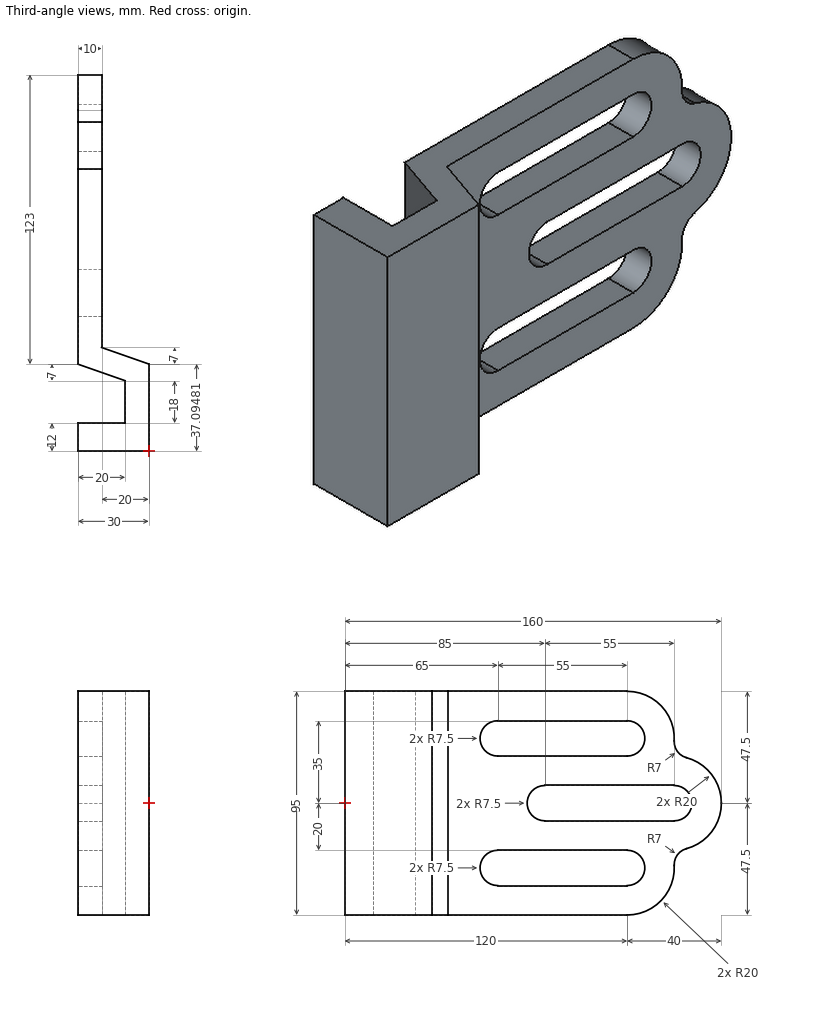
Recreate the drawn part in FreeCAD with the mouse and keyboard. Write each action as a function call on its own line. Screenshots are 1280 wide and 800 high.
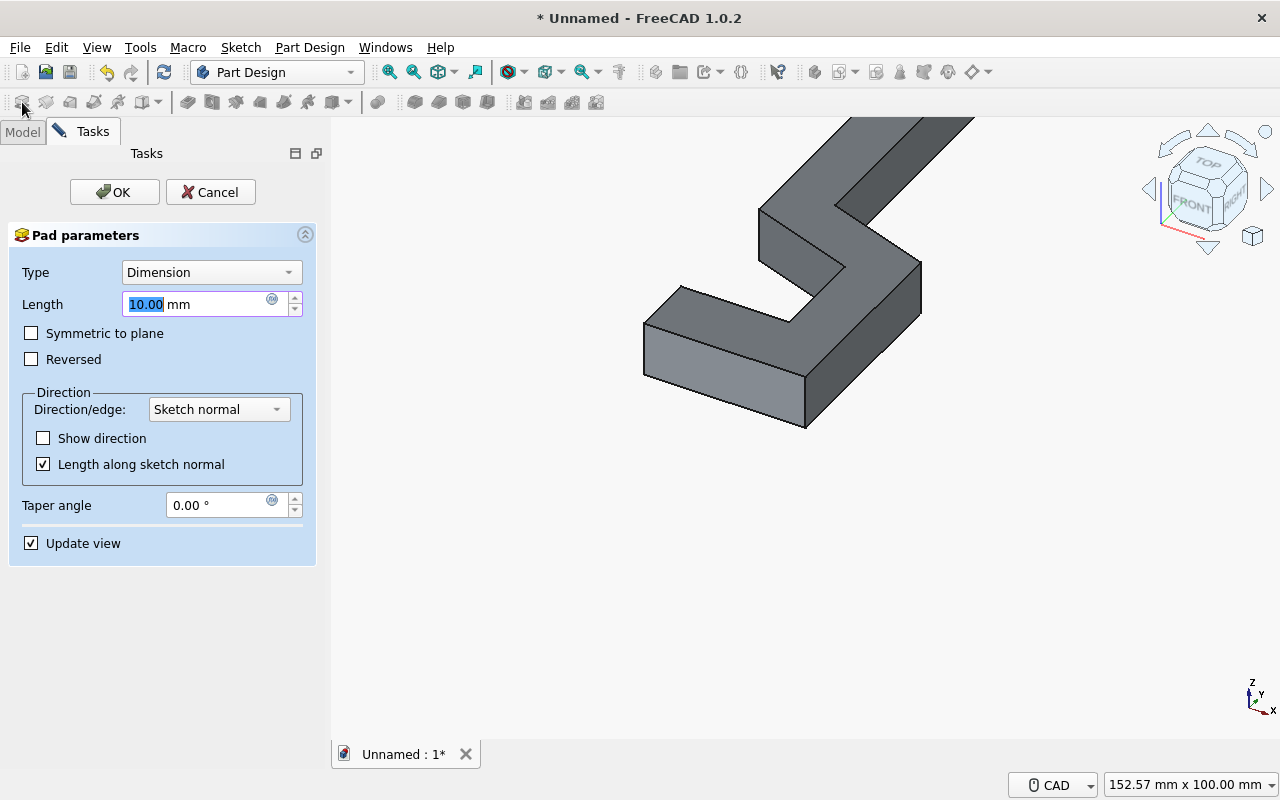
text(95)
key(Tab)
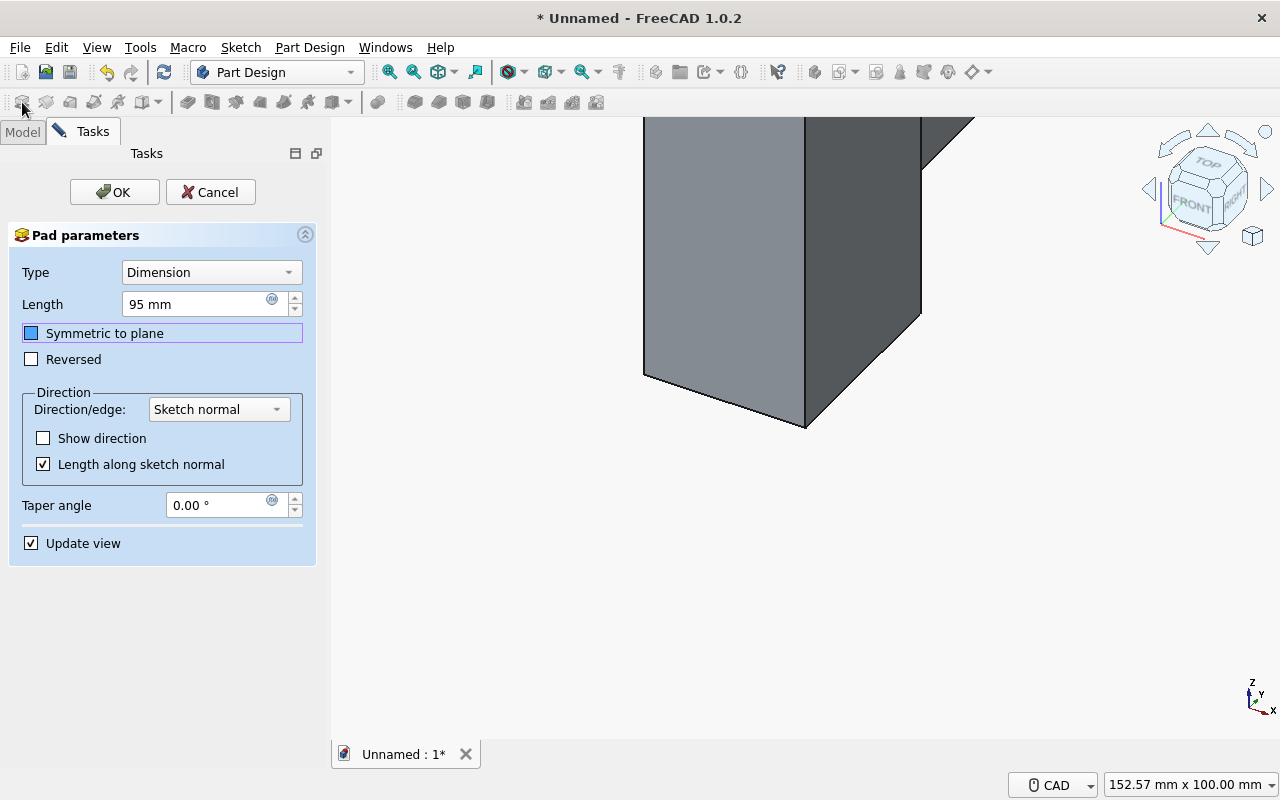
click(30, 333)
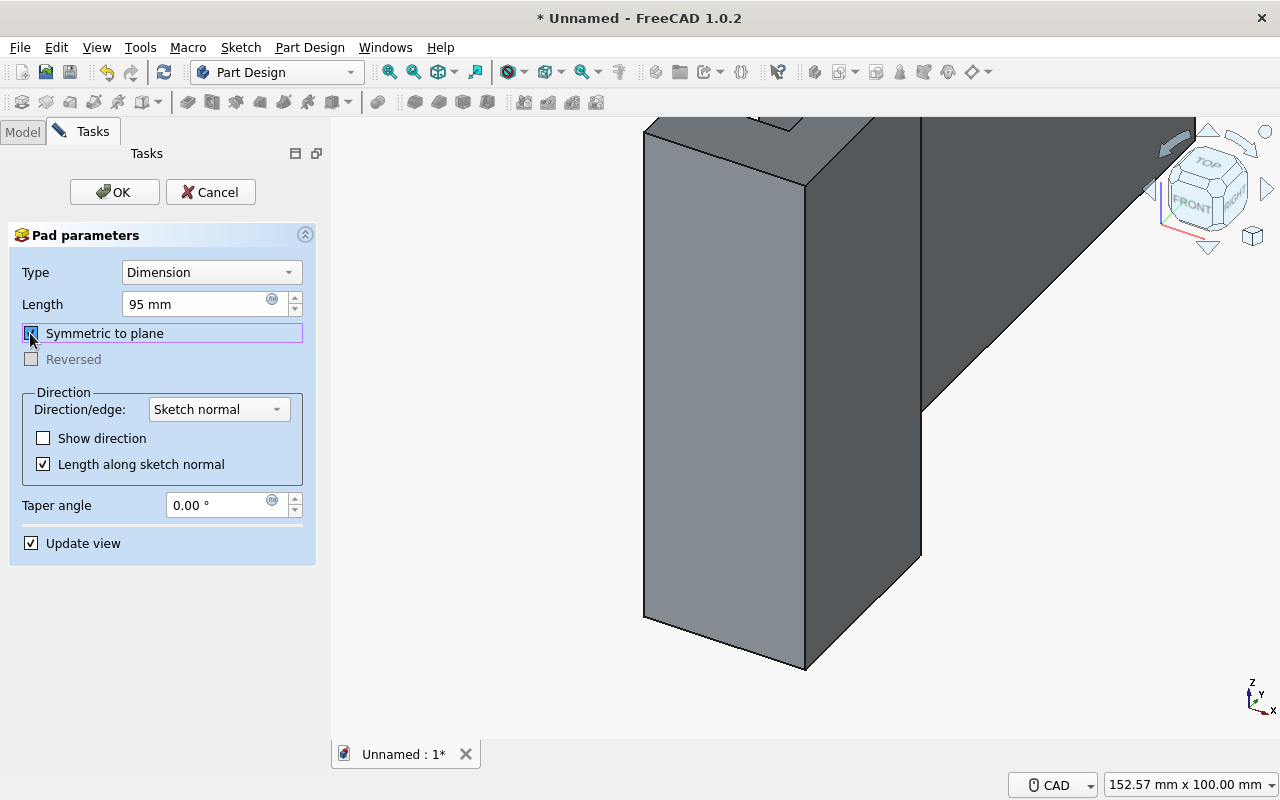
click(115, 192)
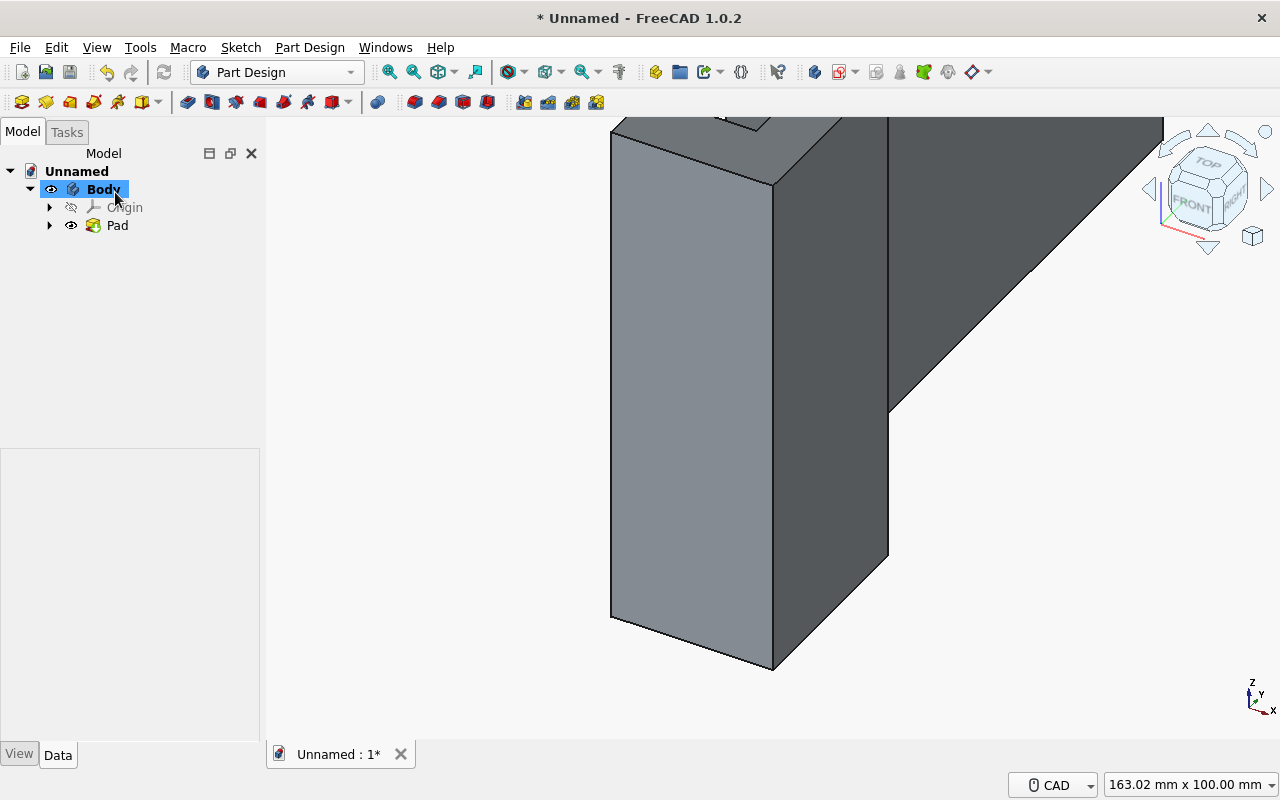
click(390, 72)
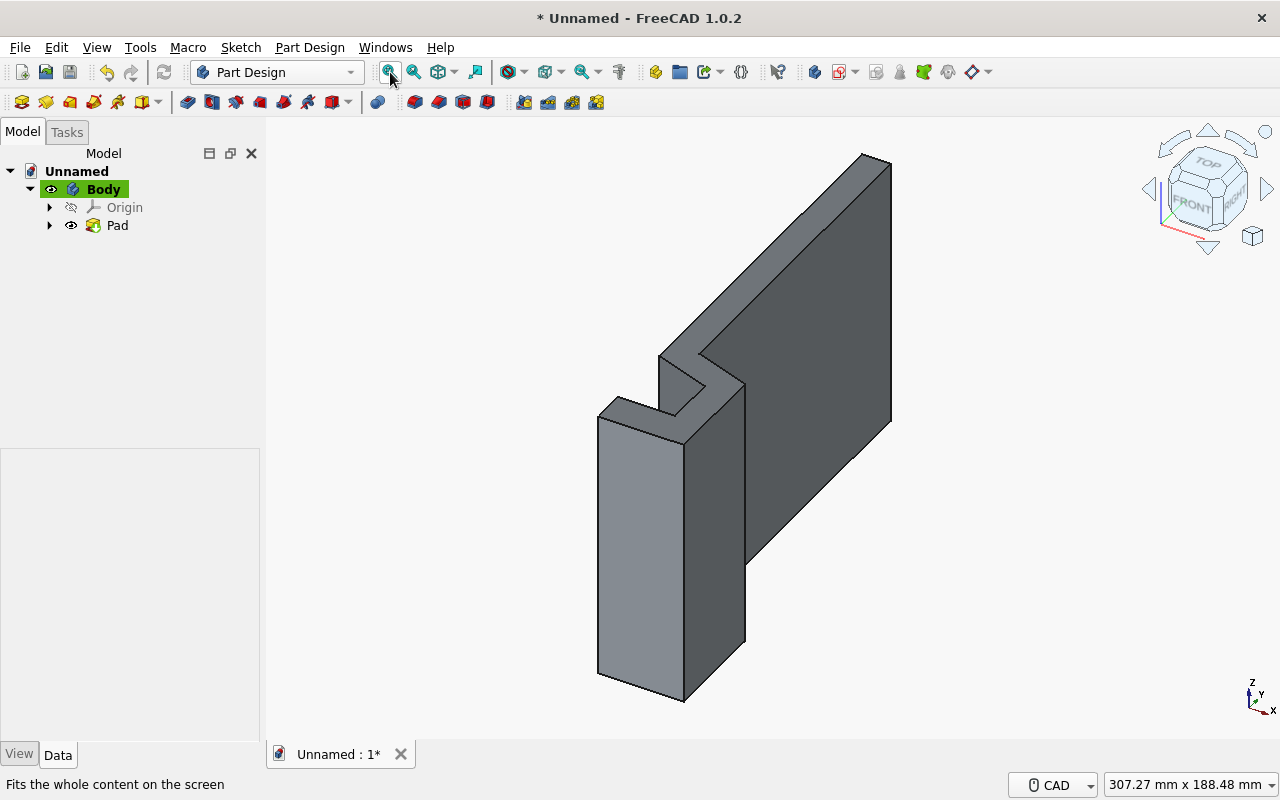
click(795, 386)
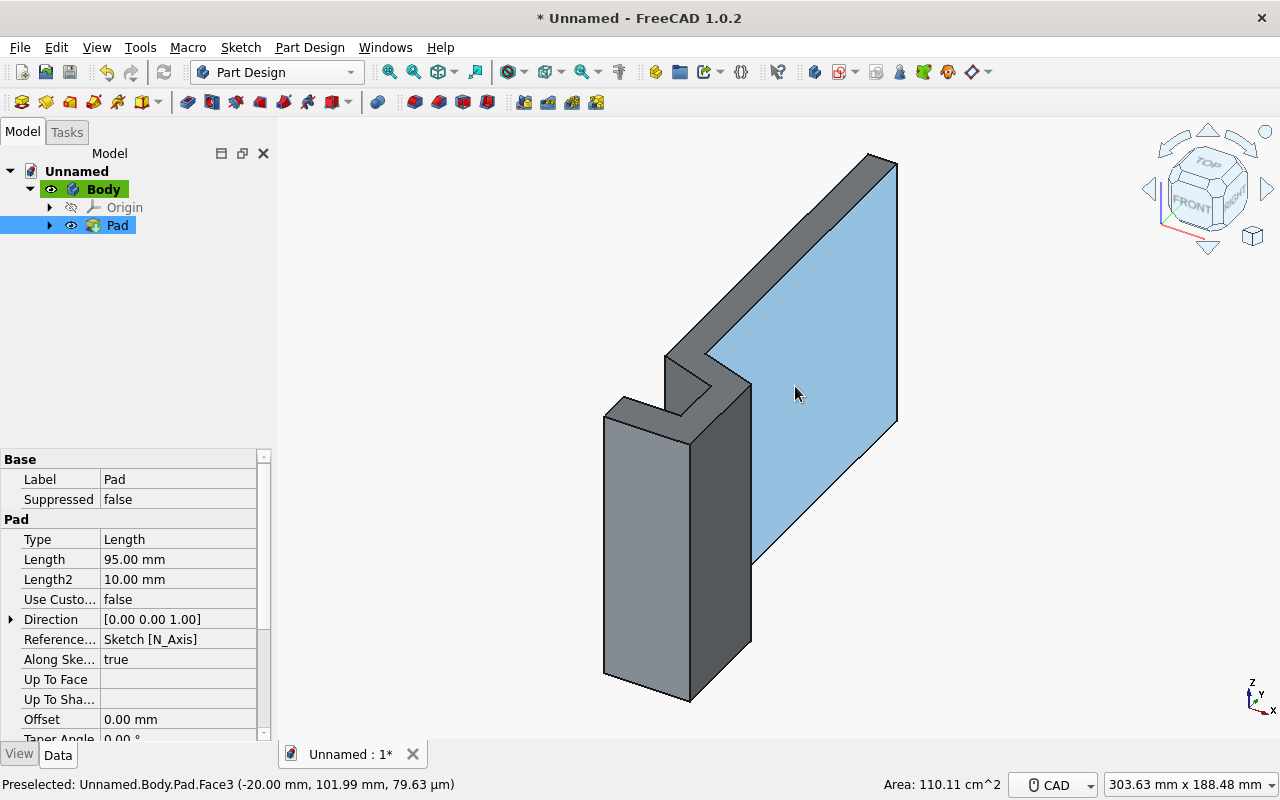
click(840, 72)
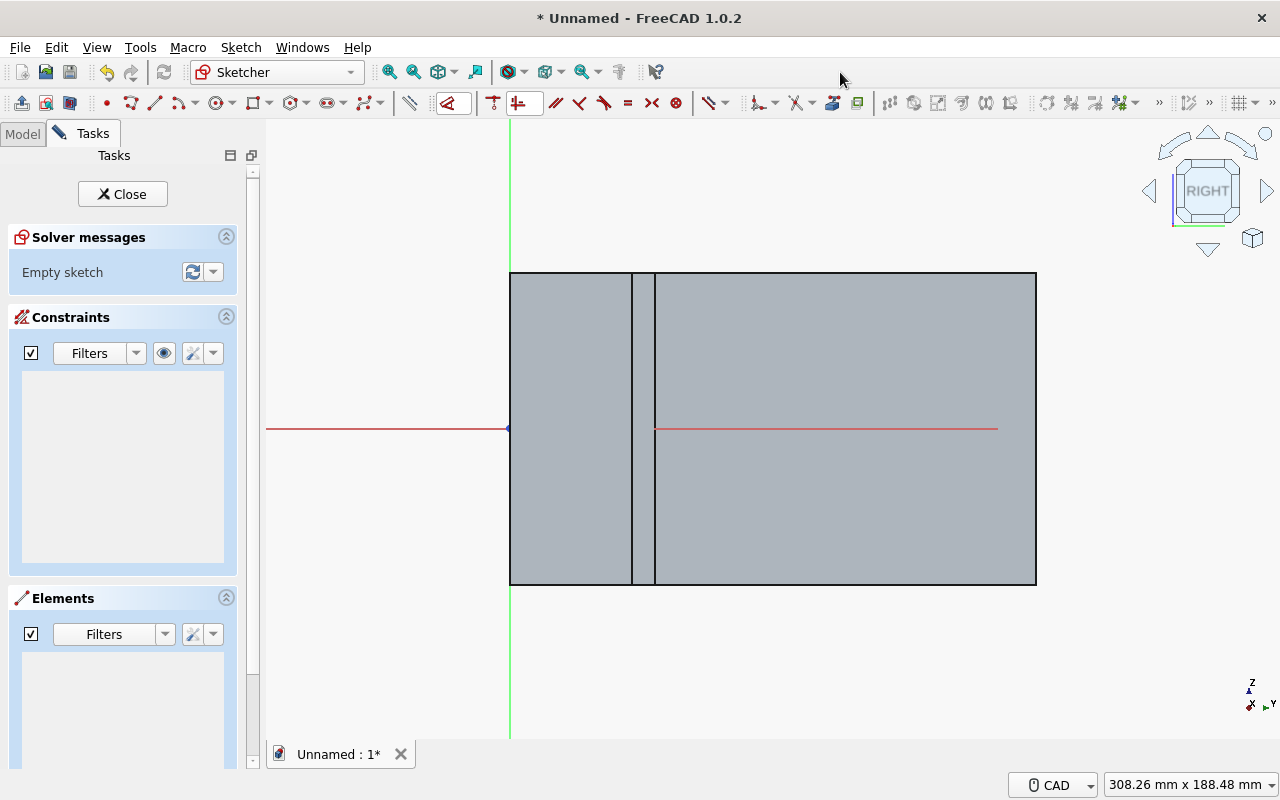
click(70, 104)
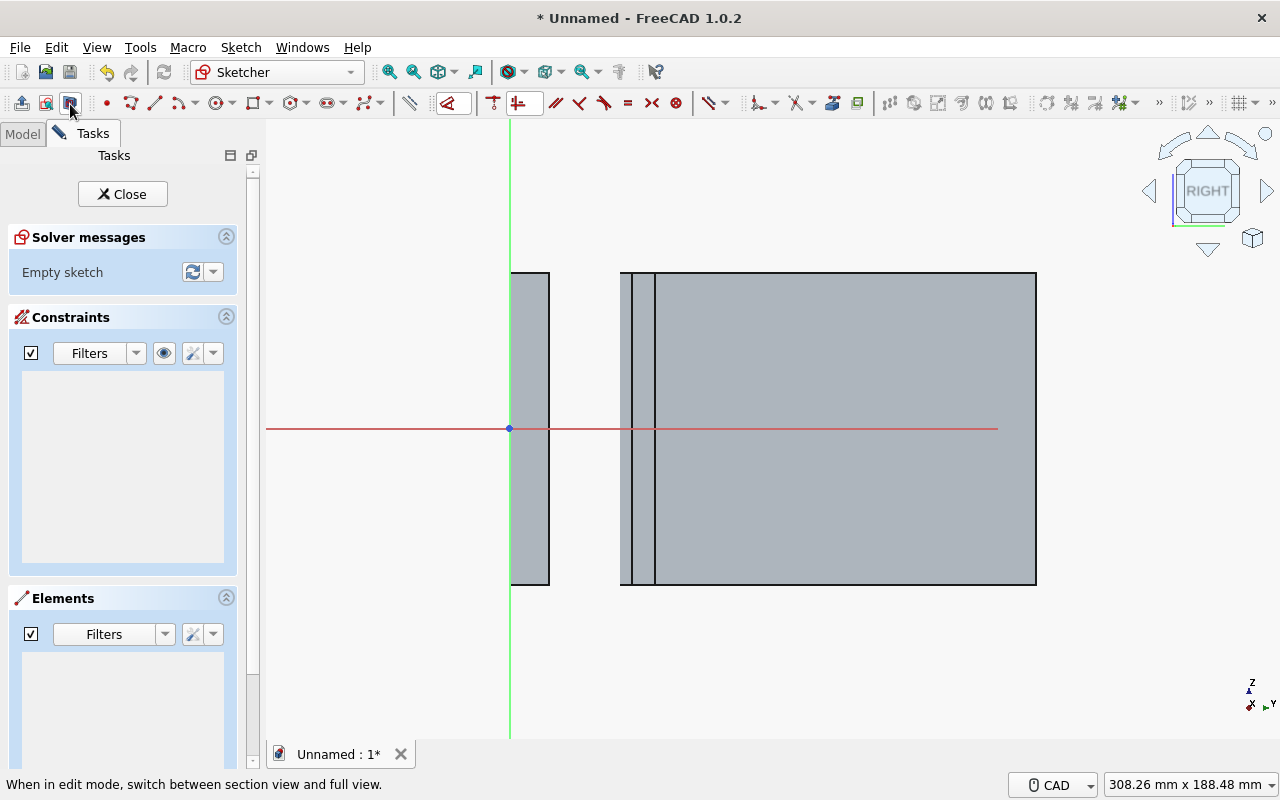
scroll(750, 254, up, 2)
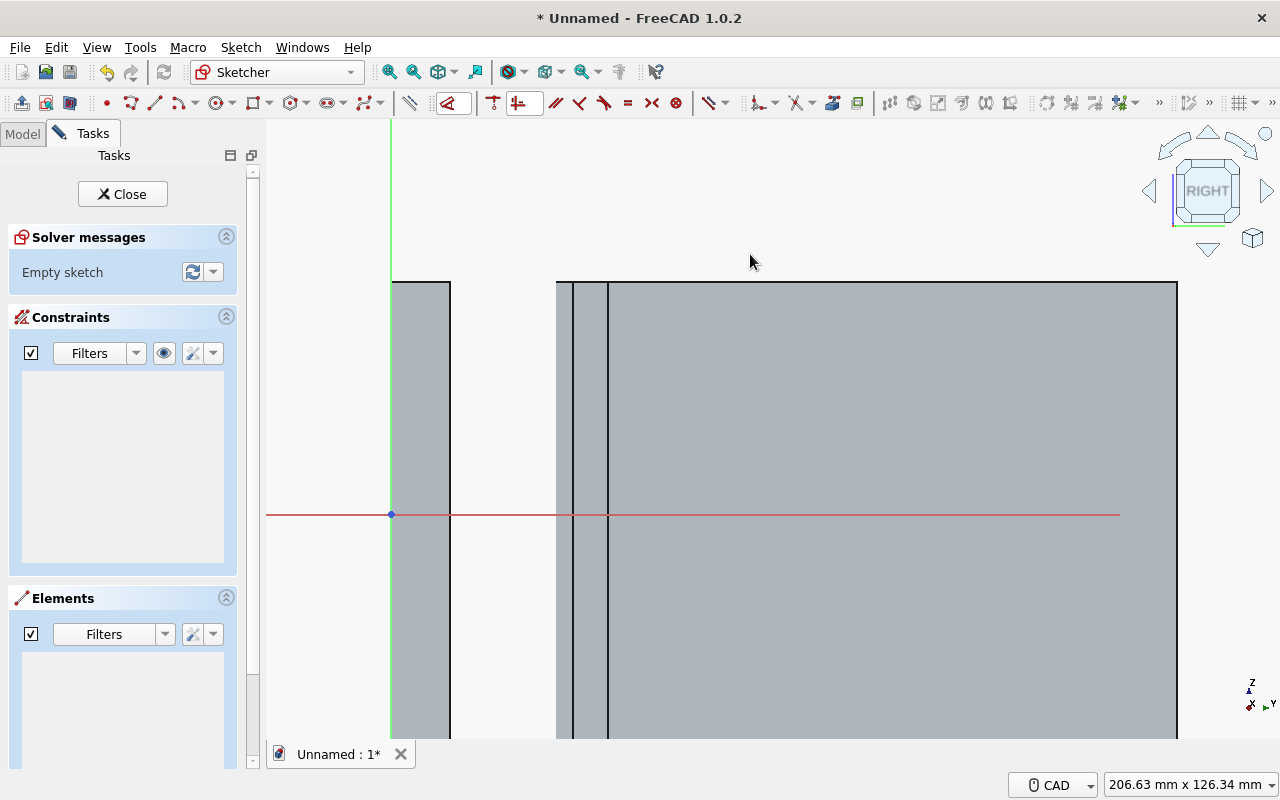
key(g)
key(s)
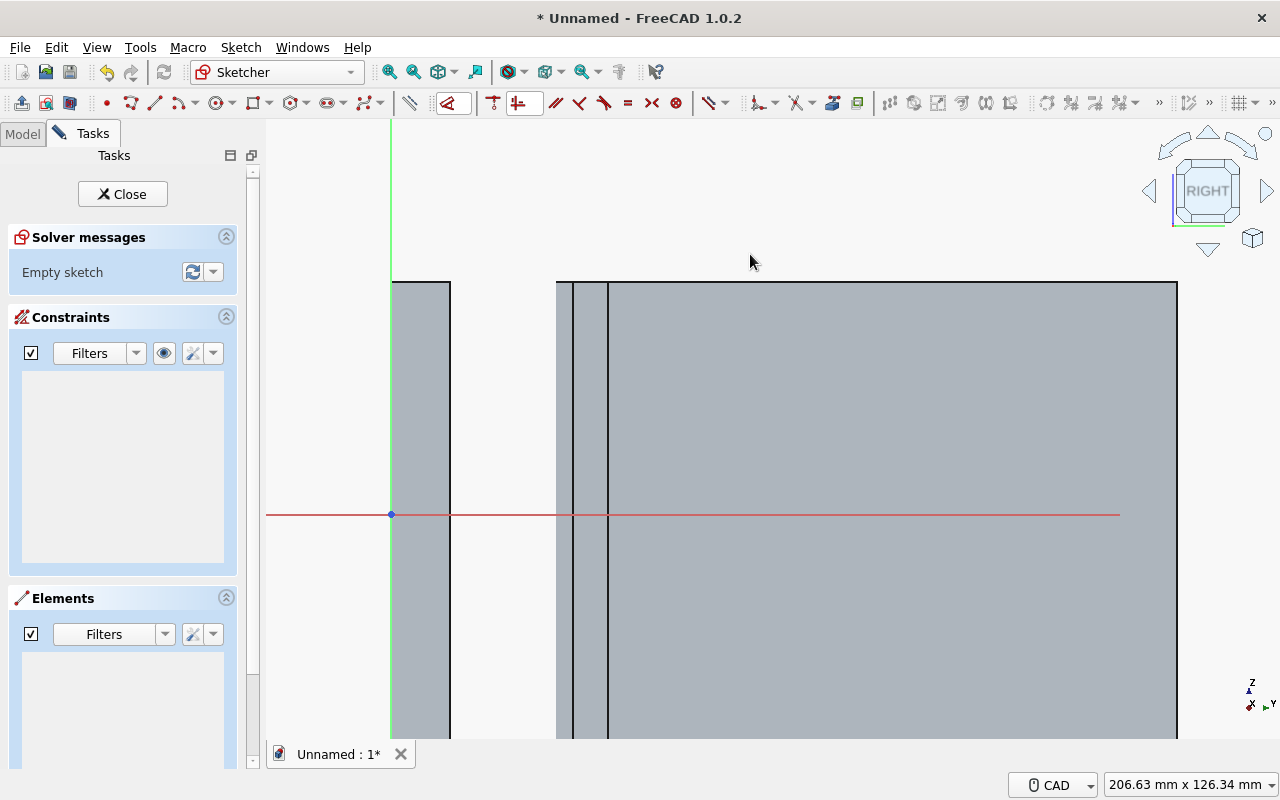
click(710, 380)